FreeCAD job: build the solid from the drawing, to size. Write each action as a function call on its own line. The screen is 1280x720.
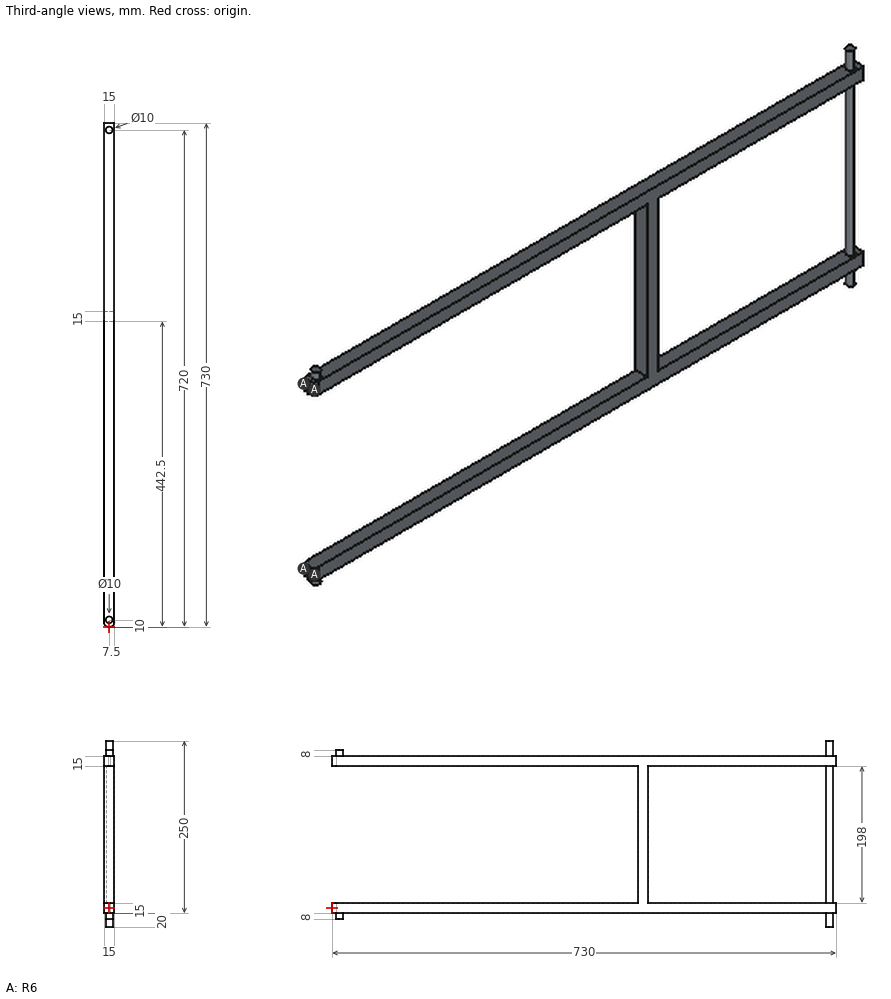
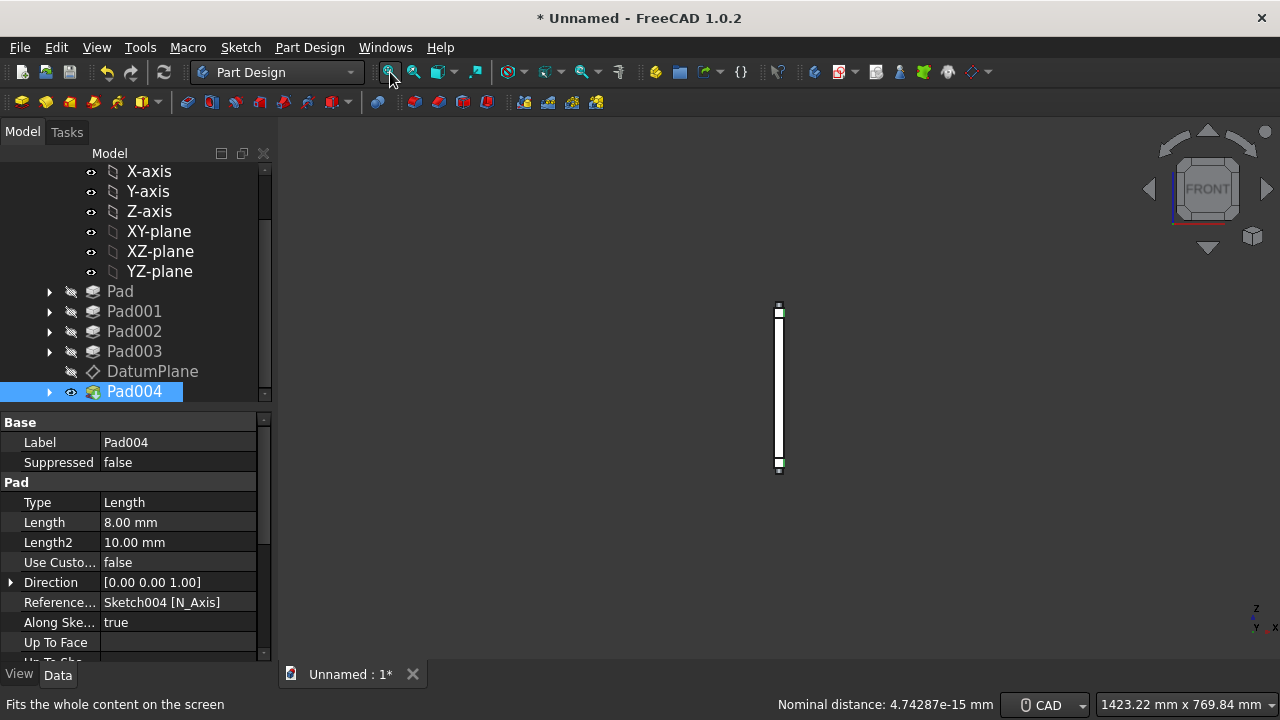
click(774, 466, ctrl)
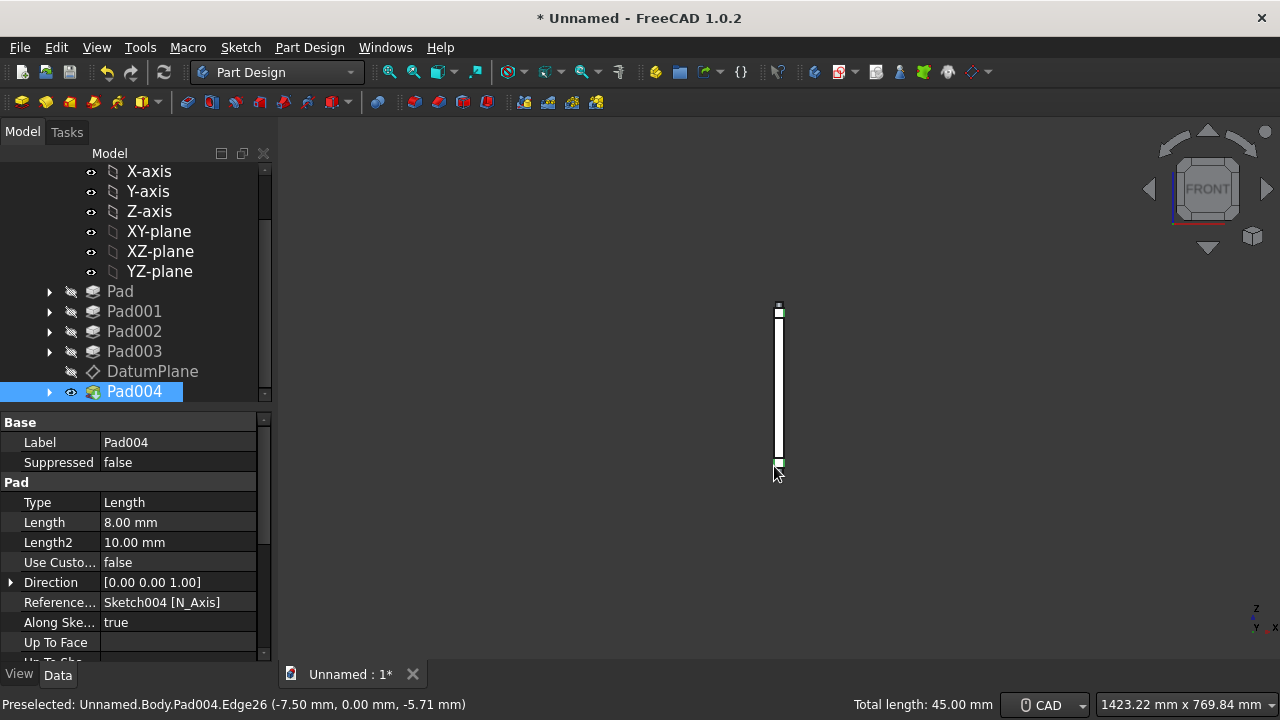
scroll(774, 312, up, 7)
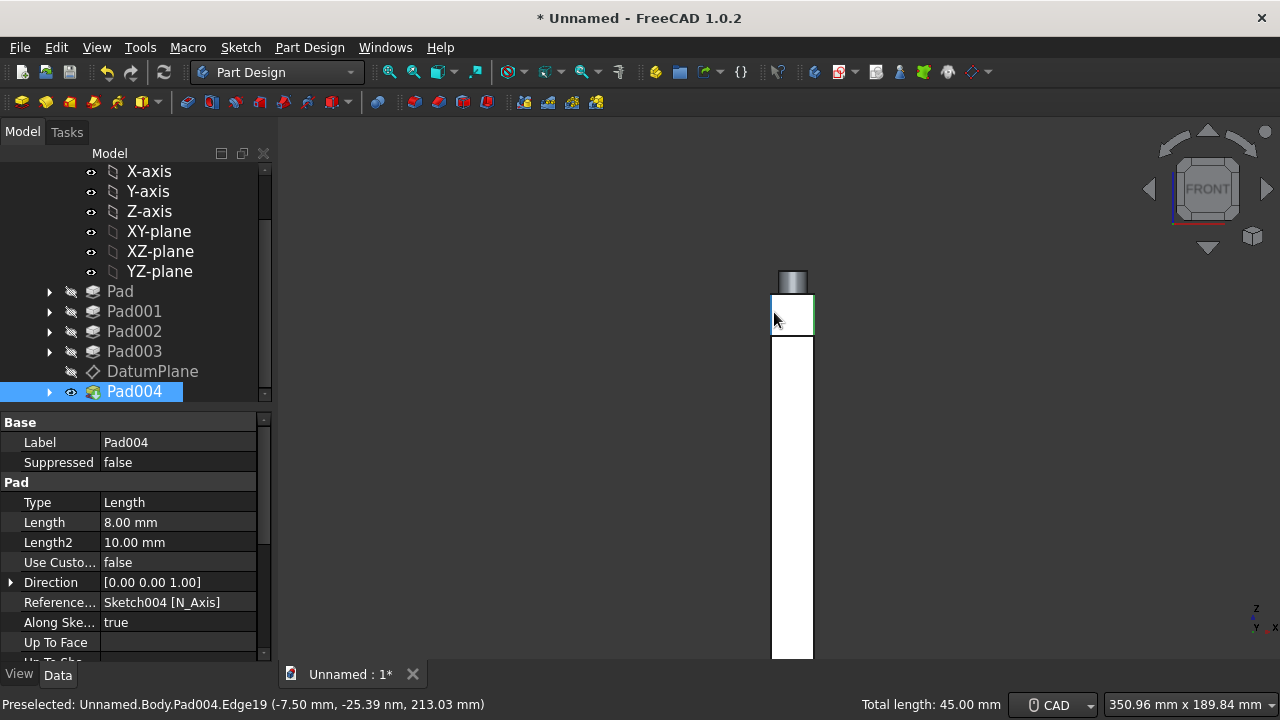
click(771, 323, ctrl)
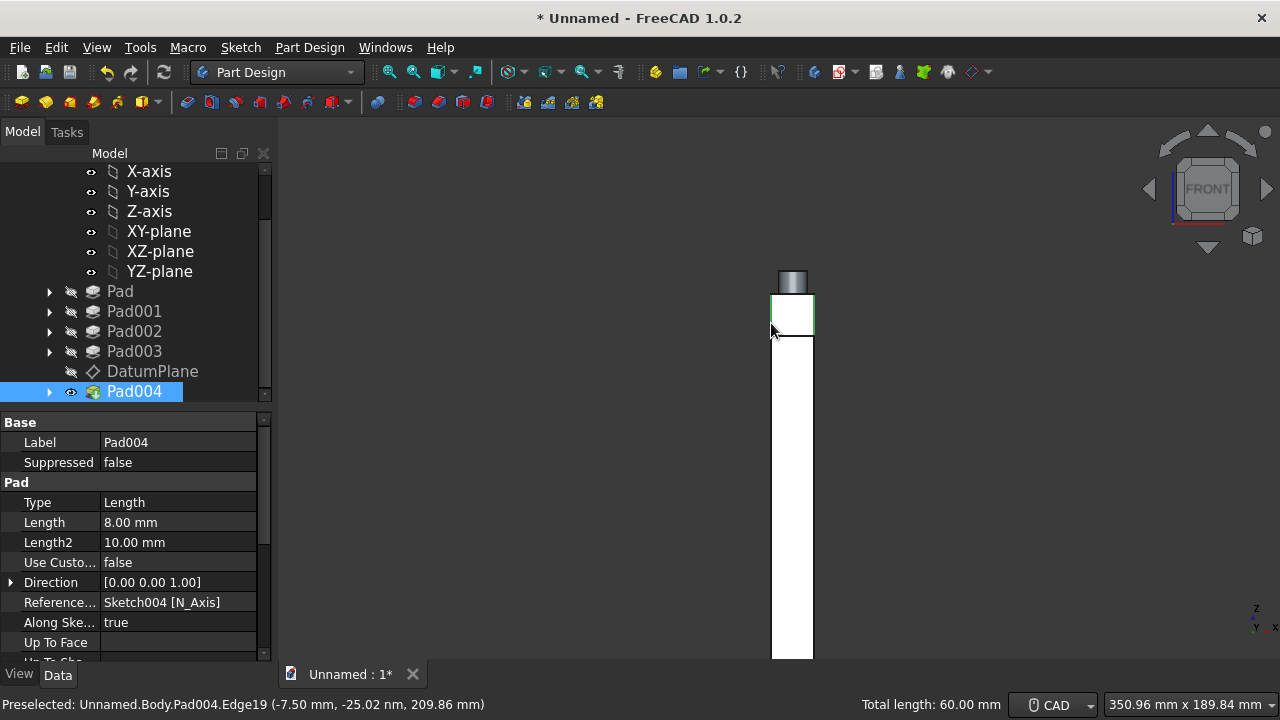
click(416, 102)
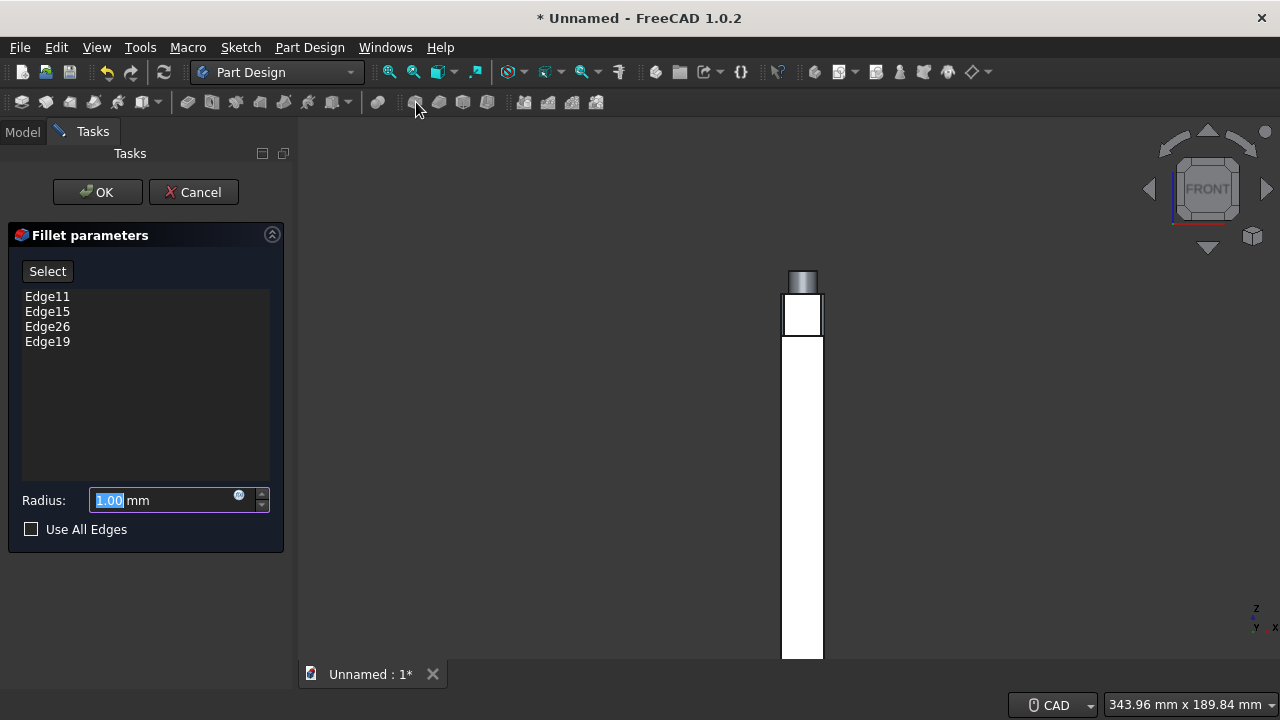
text(6)
key(Tab)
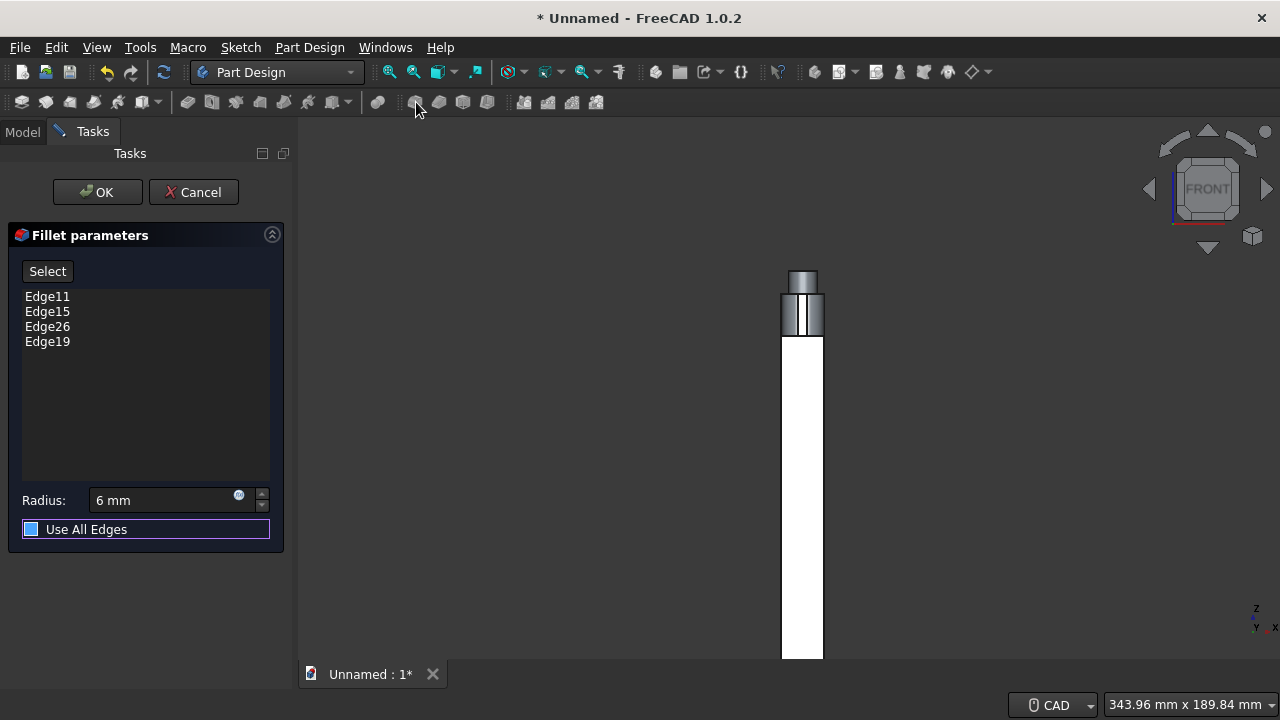
click(98, 192)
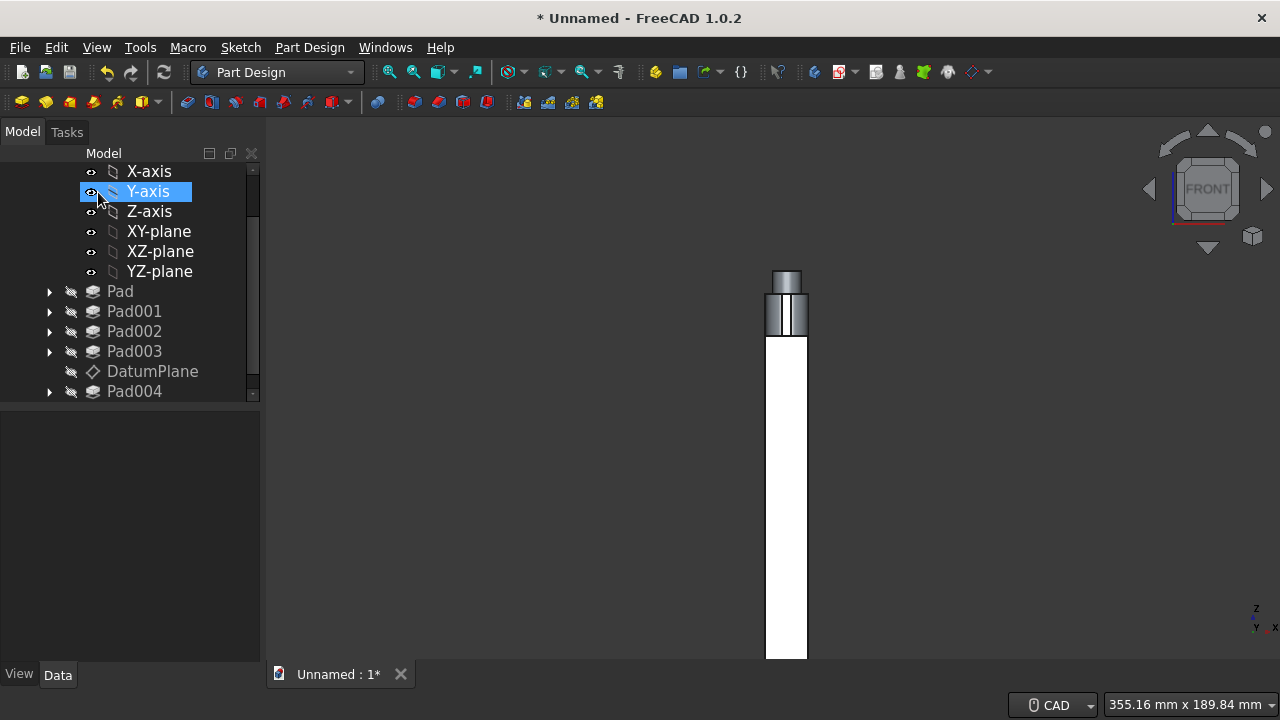
click(390, 72)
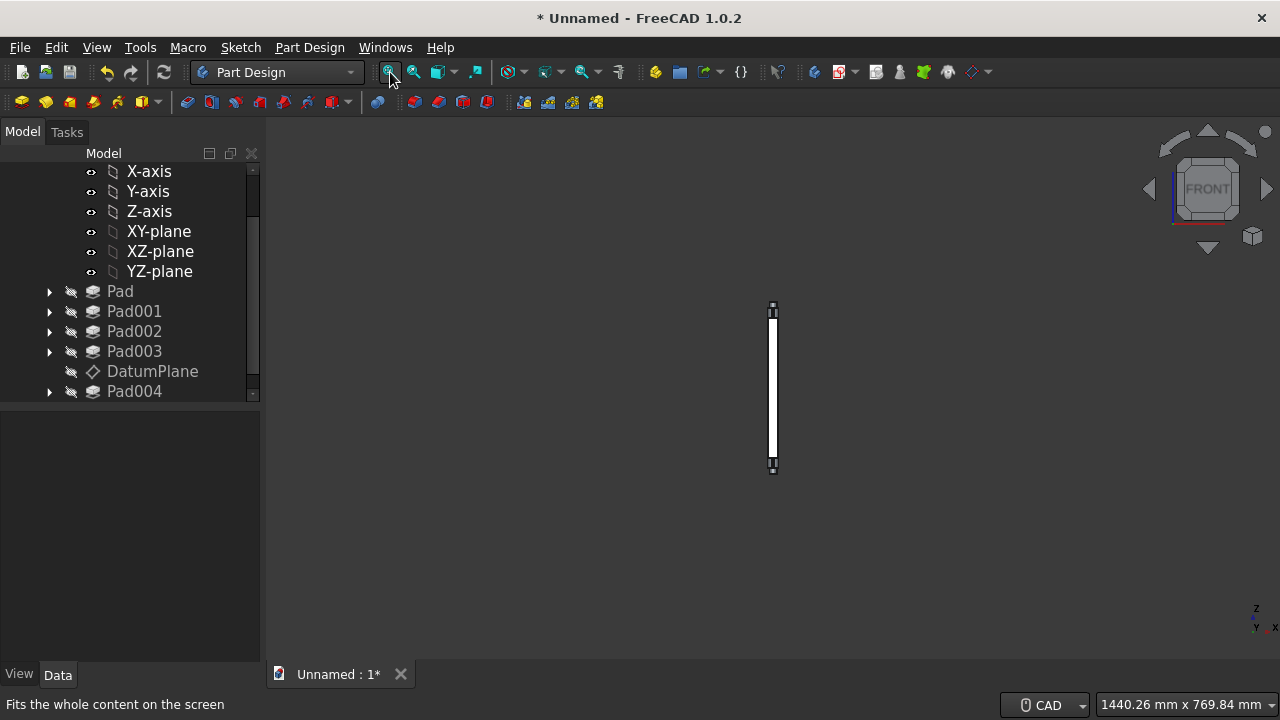
key(5)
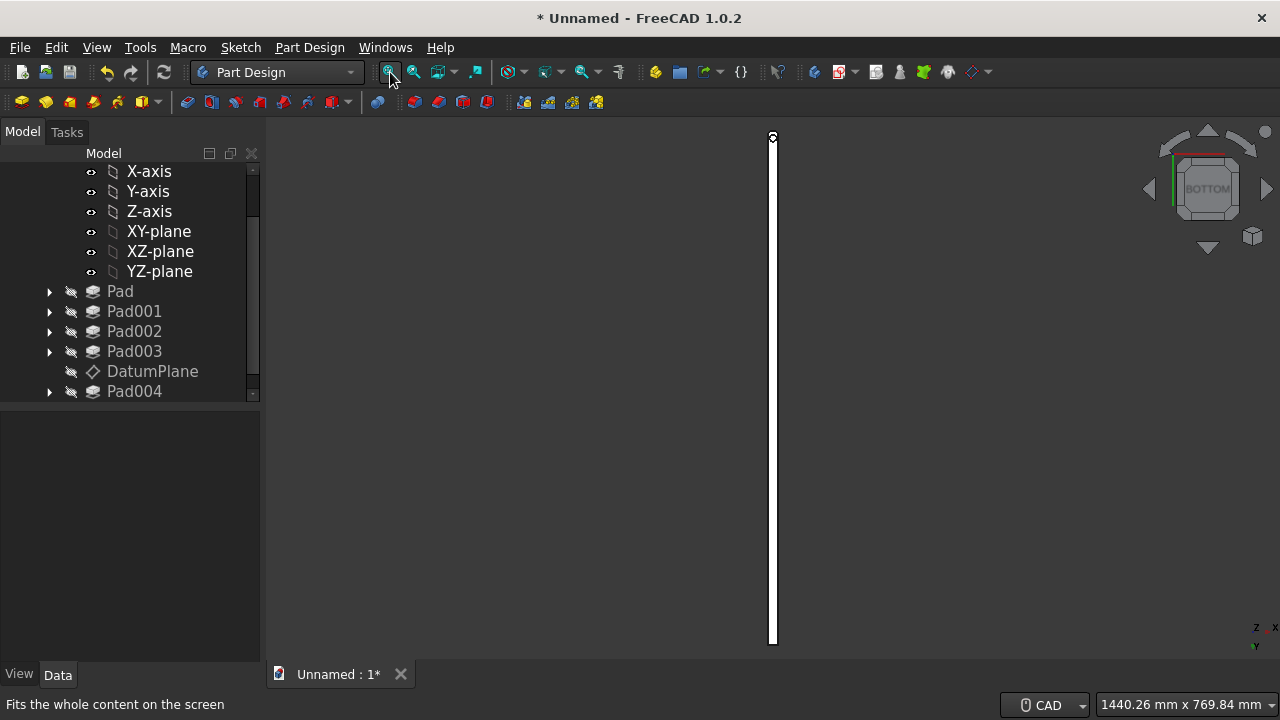
scroll(773, 607, up, 5)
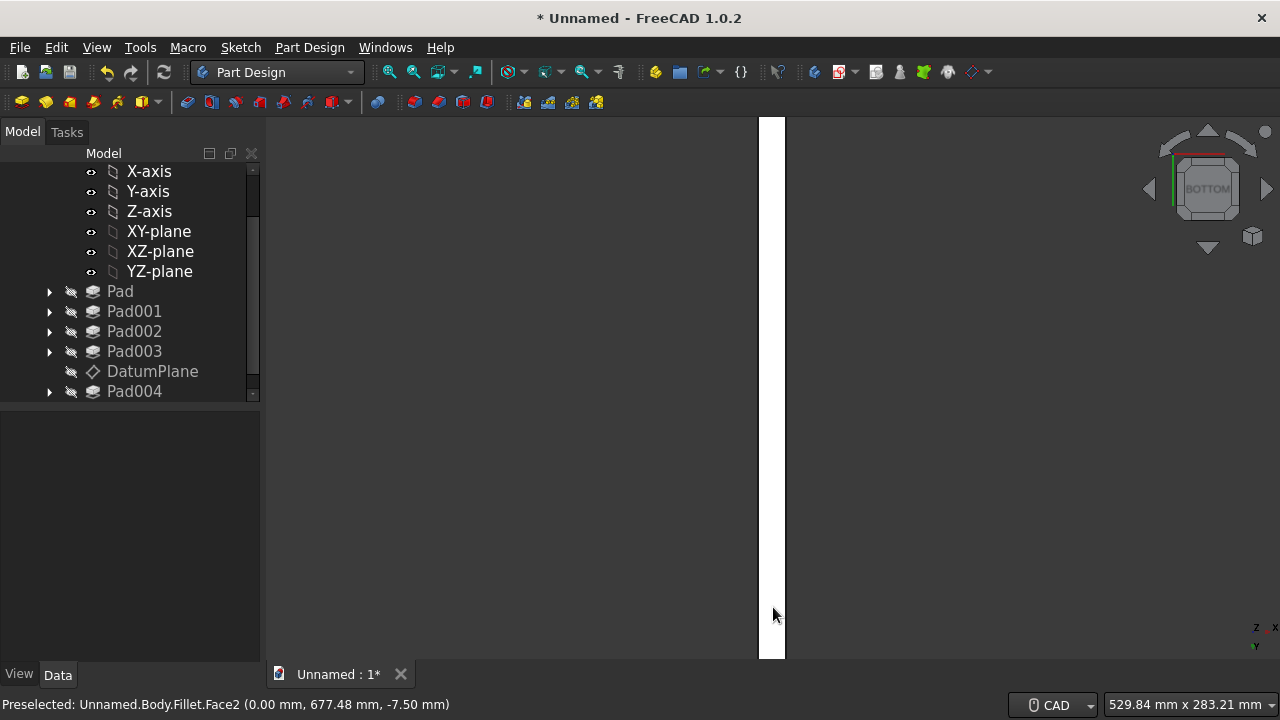
click(772, 608)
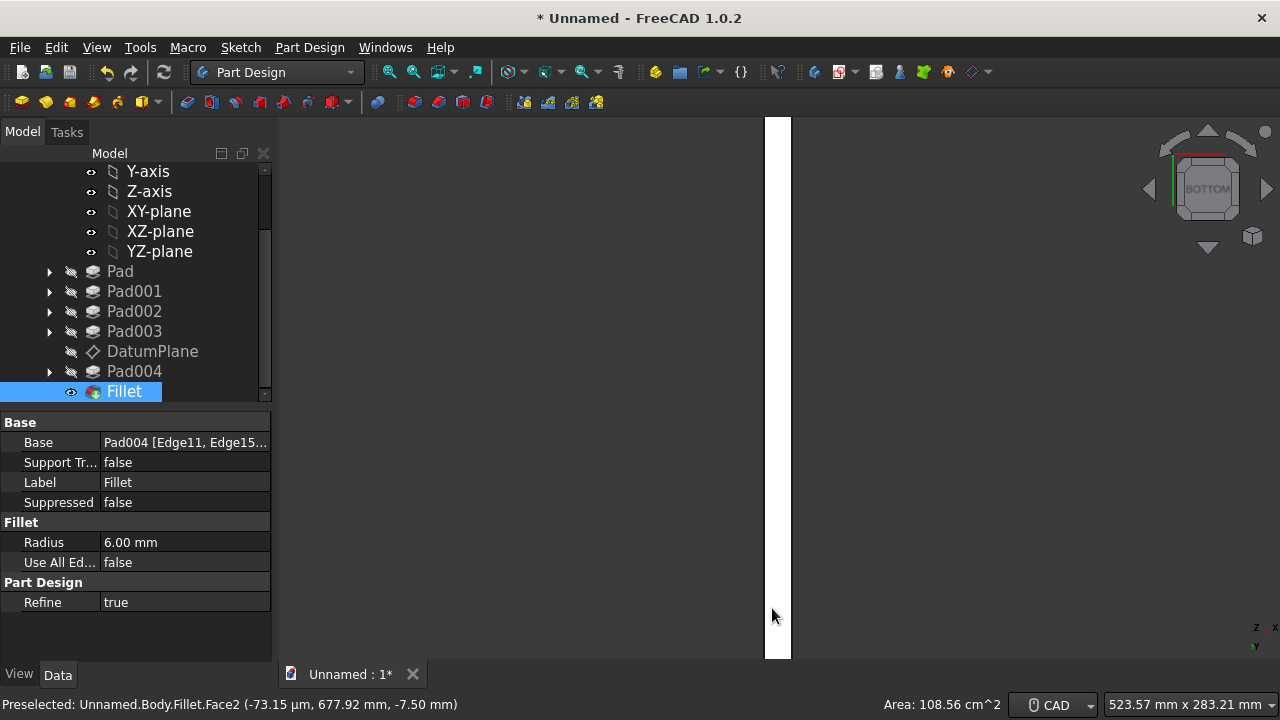
click(840, 72)